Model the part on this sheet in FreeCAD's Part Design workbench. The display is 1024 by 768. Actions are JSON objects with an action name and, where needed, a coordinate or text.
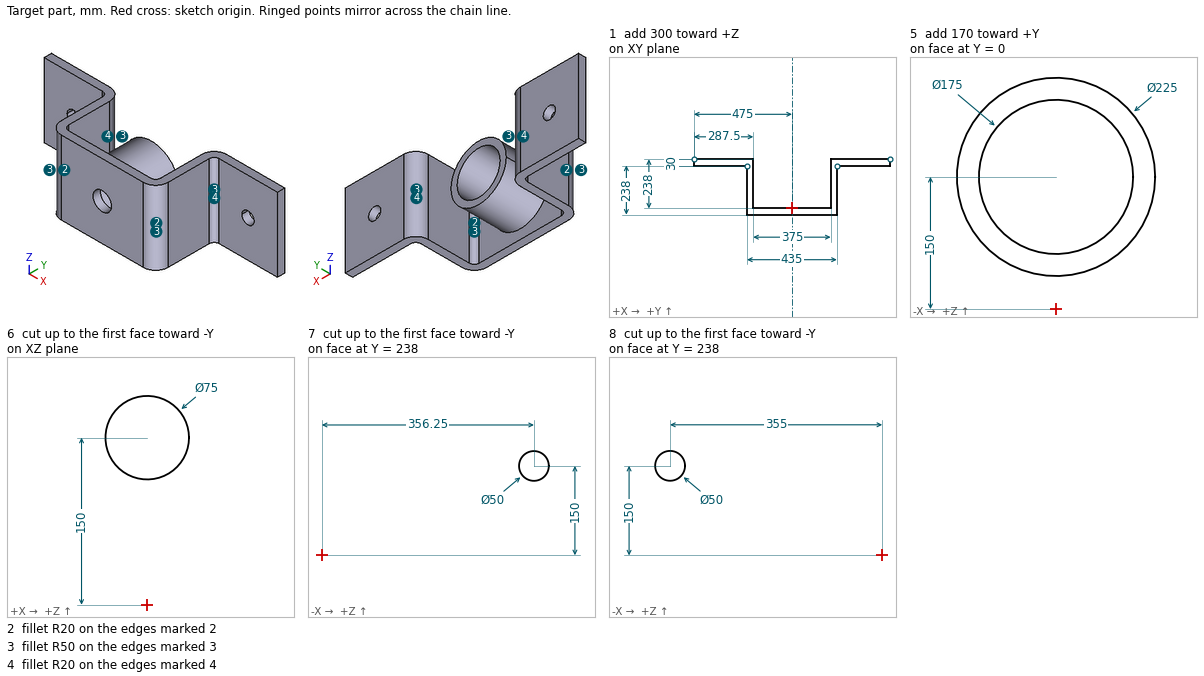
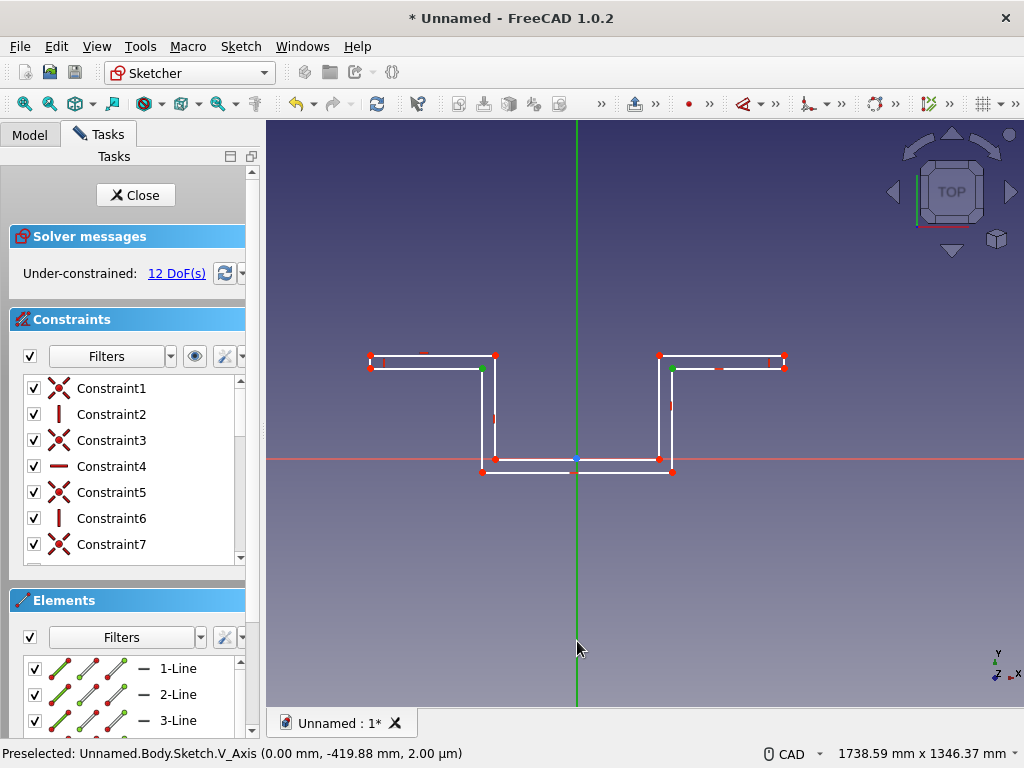
{"action": "key", "text": "s"}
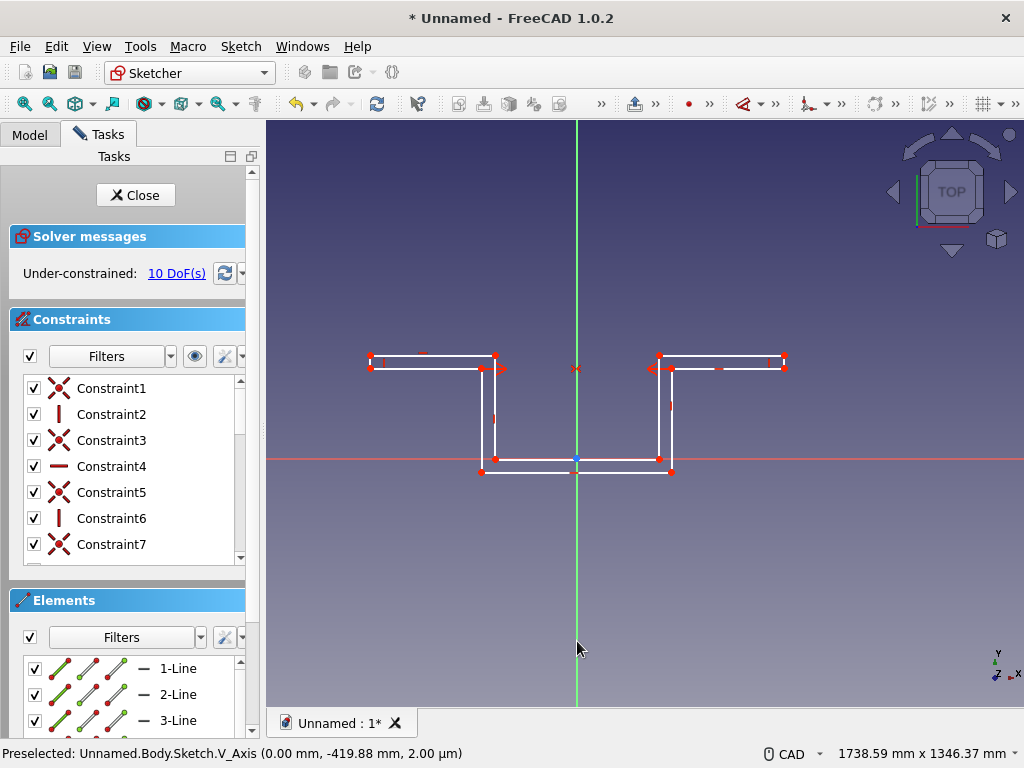
{"action": "left_click", "coordinate": [370, 356]}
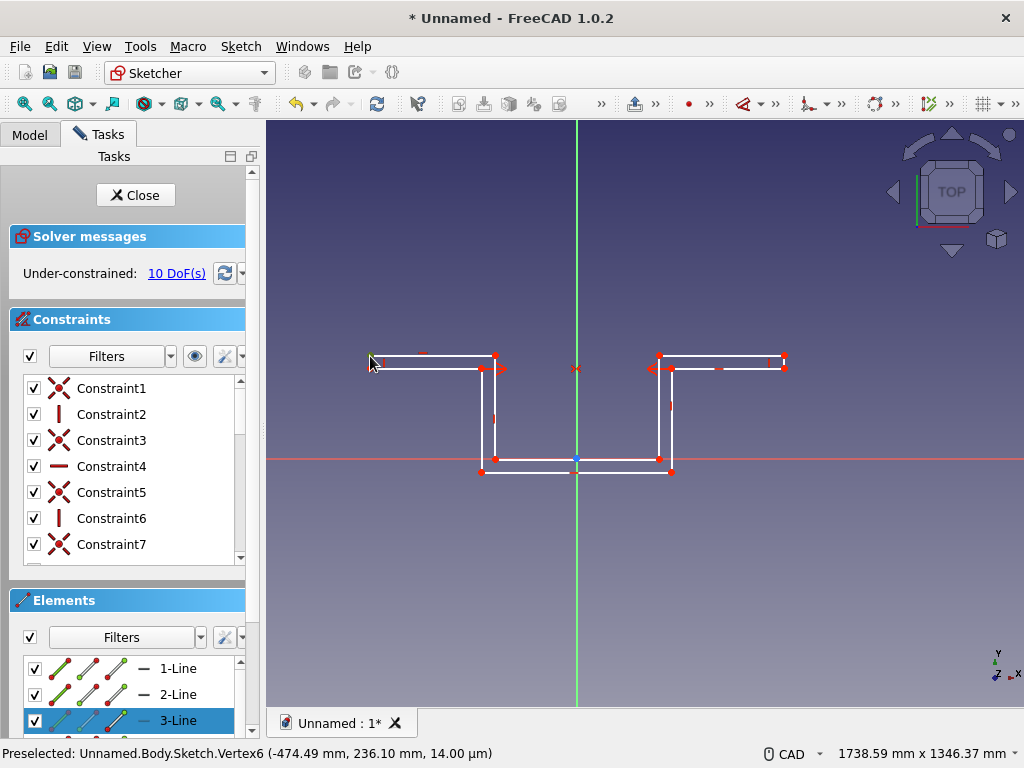
{"action": "left_click", "coordinate": [784, 356]}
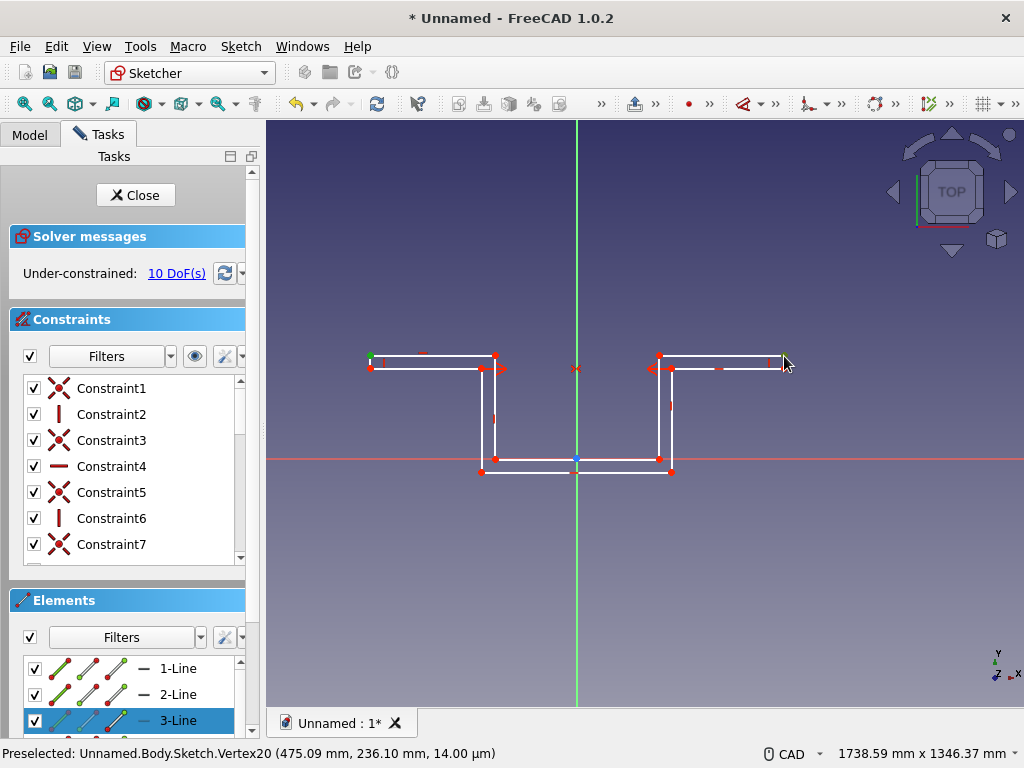
{"action": "left_click", "coordinate": [577, 641]}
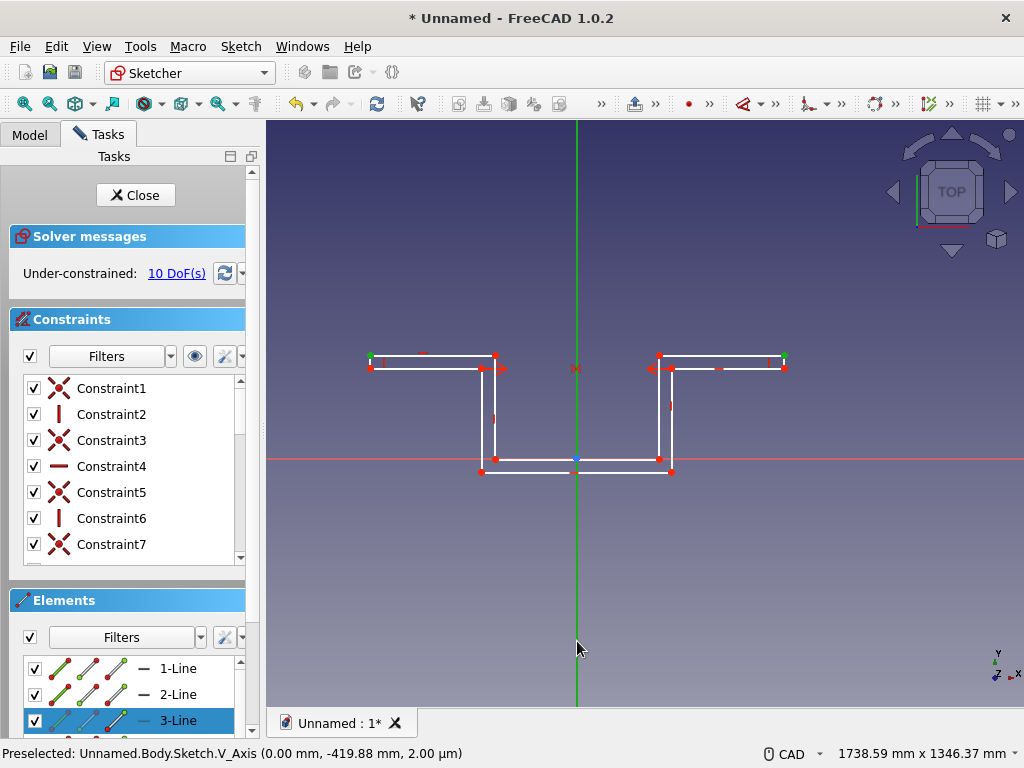
{"action": "key", "text": "s"}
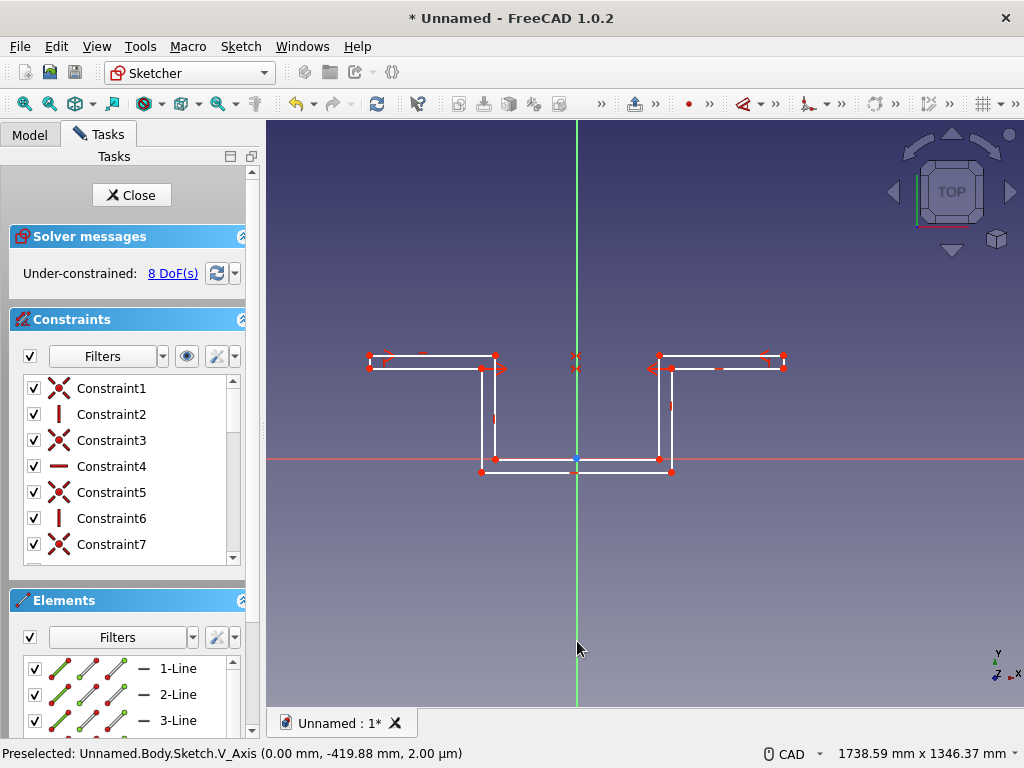
{"action": "left_click", "coordinate": [659, 460]}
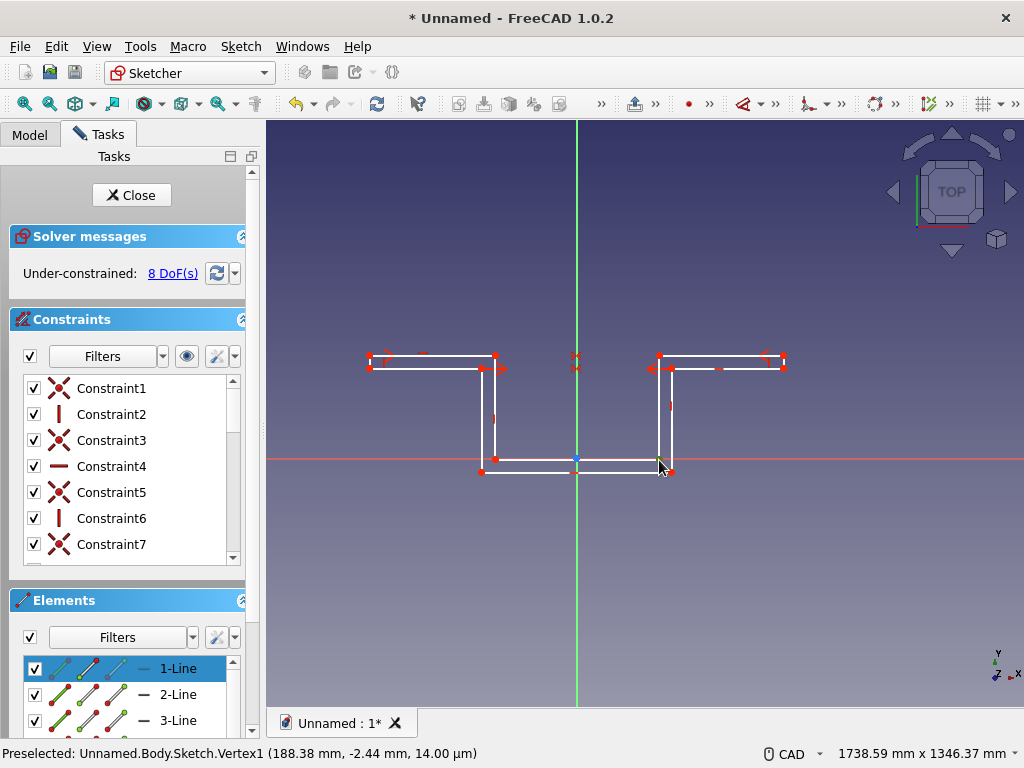
{"action": "left_click", "coordinate": [334, 459]}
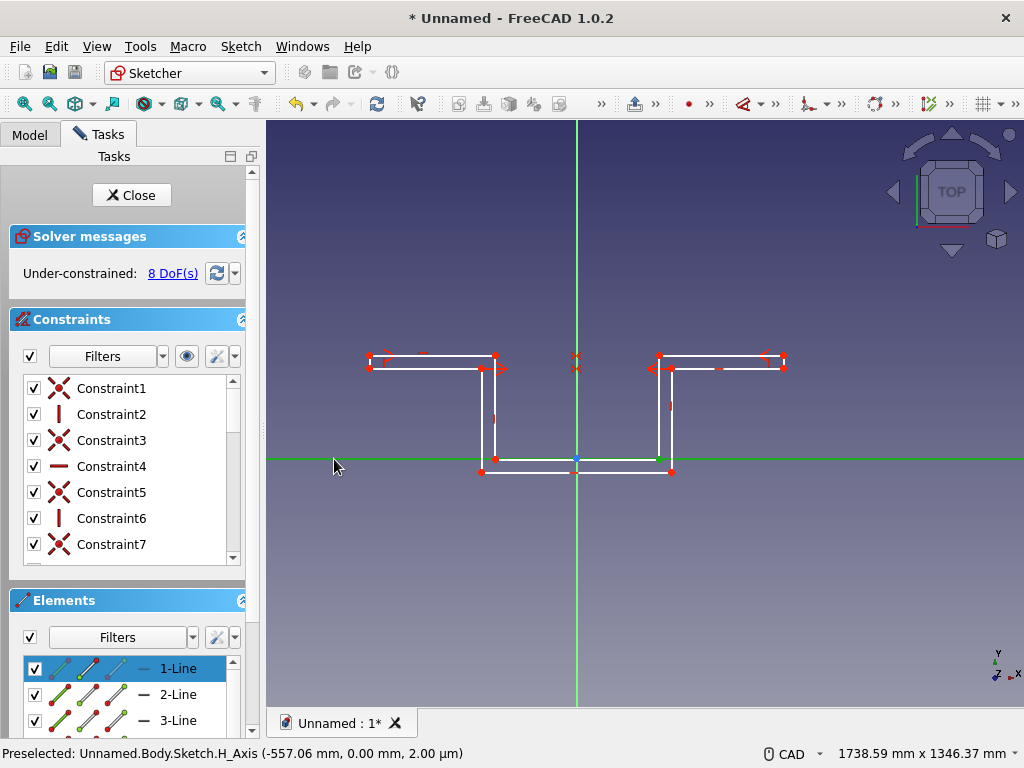
{"action": "key", "text": "c"}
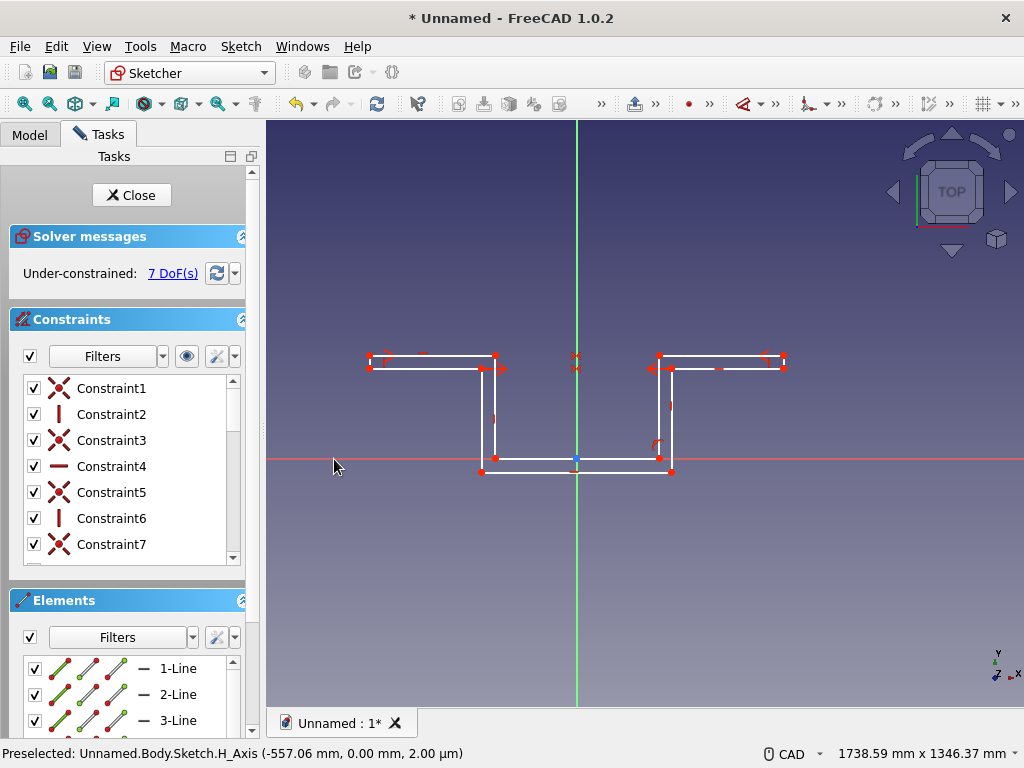
{"action": "key", "text": "d"}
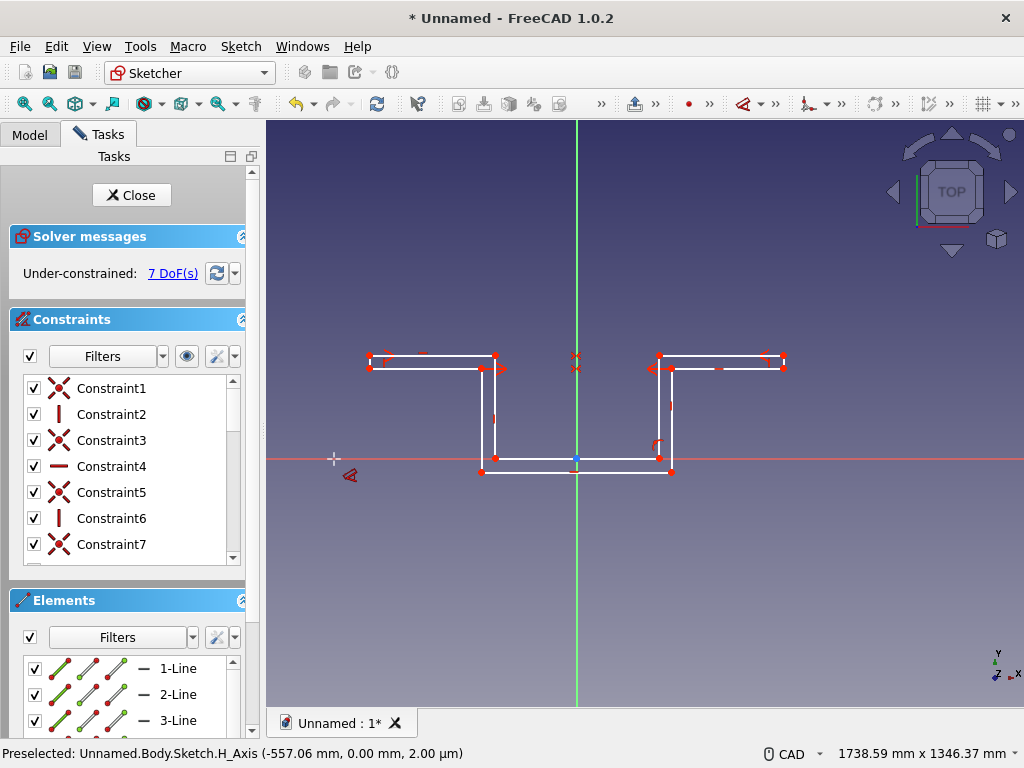
{"action": "scroll", "coordinate": [370, 363], "scroll_direction": "up", "scroll_amount": 6}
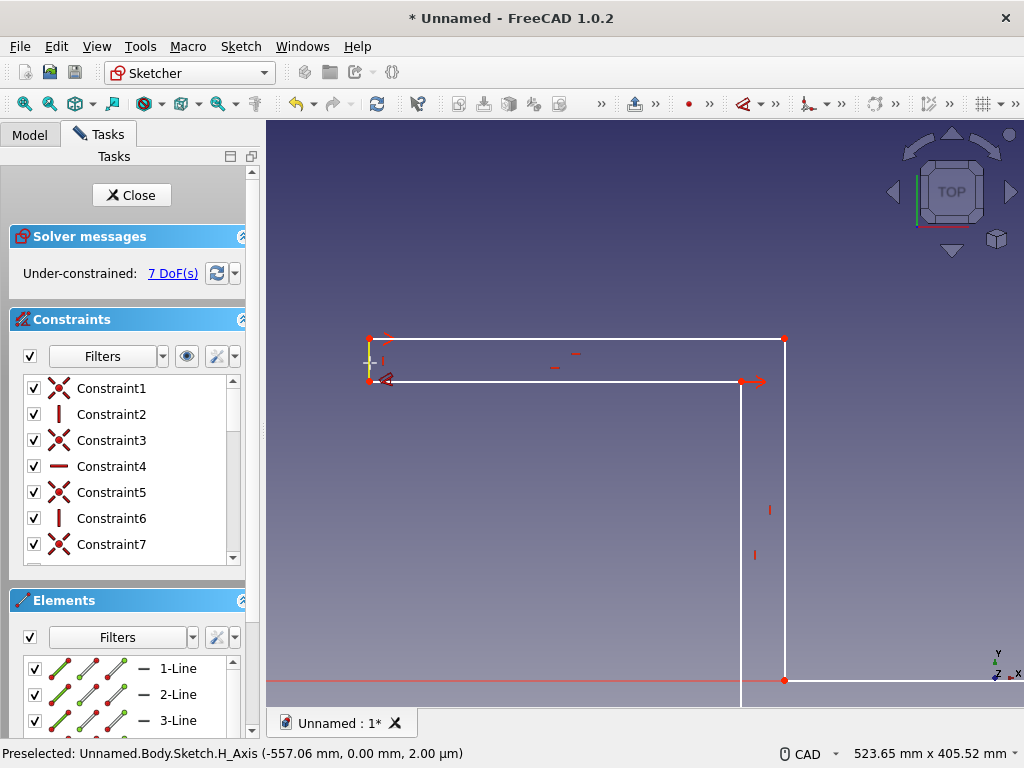
{"action": "left_click", "coordinate": [369, 360]}
{"action": "left_click", "coordinate": [335, 360]}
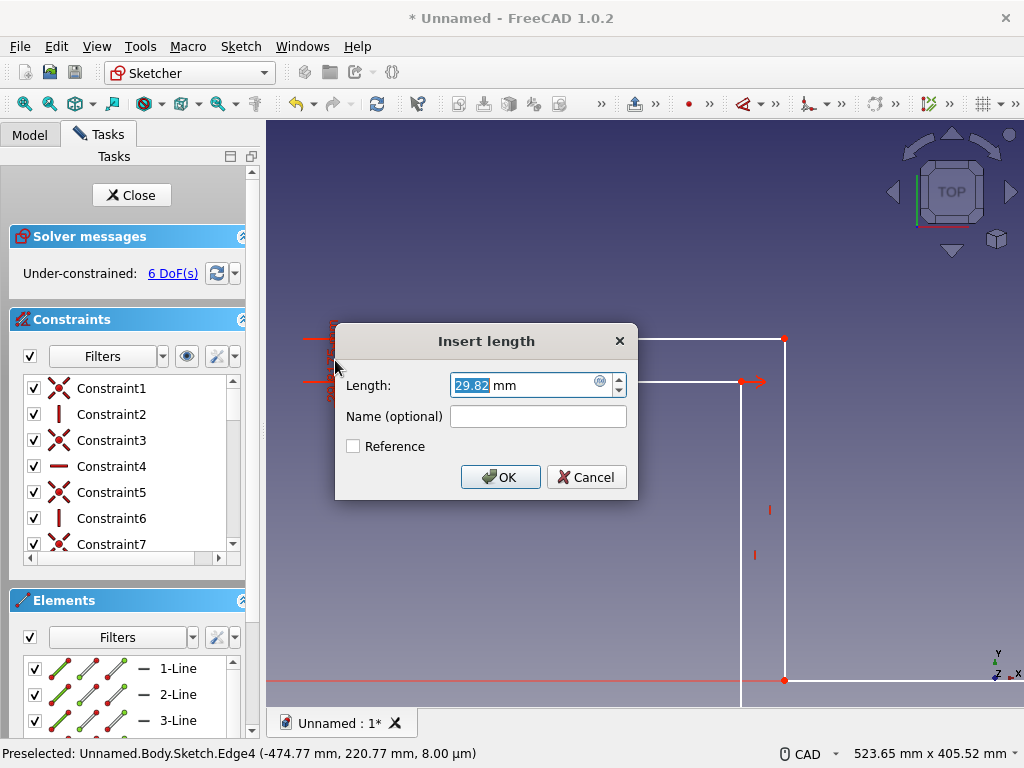
{"action": "type", "text": "30"}
{"action": "key", "text": "Return"}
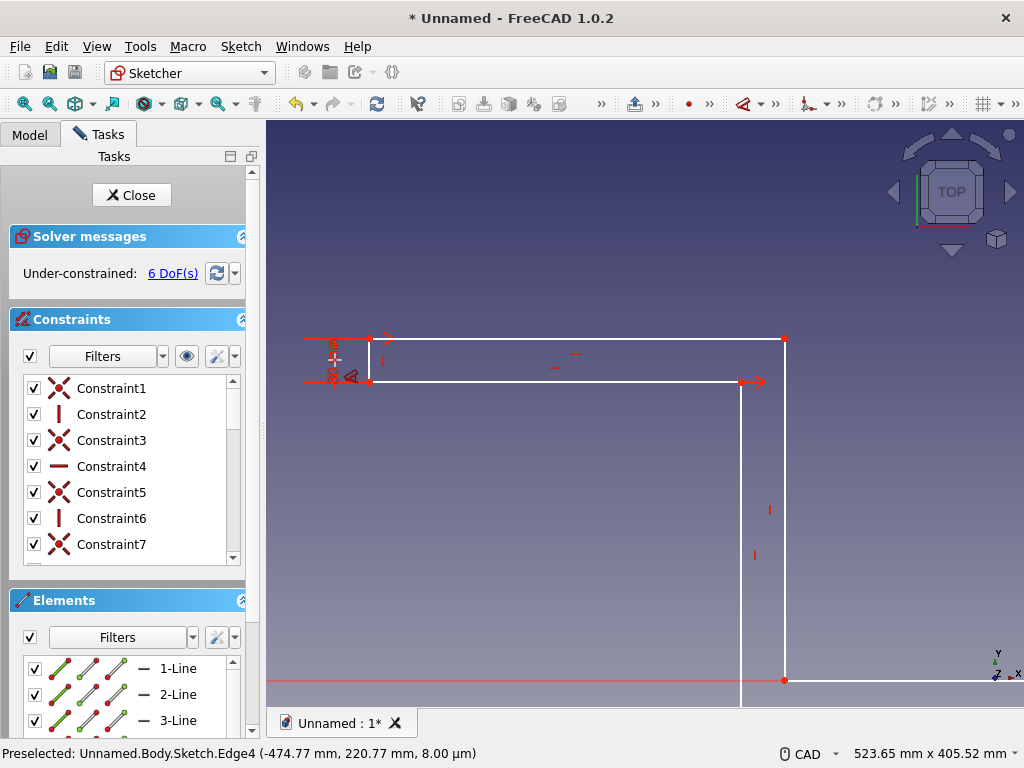
{"action": "scroll", "coordinate": [370, 363], "scroll_direction": "down", "scroll_amount": 6}